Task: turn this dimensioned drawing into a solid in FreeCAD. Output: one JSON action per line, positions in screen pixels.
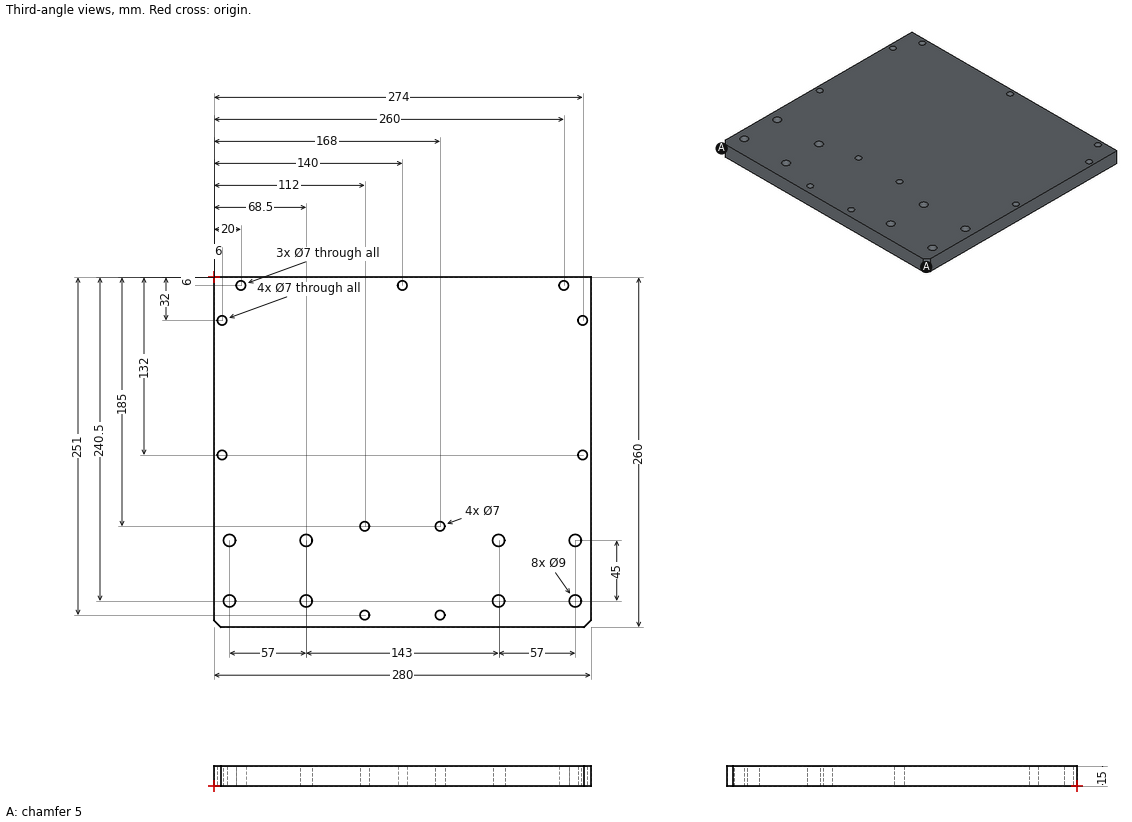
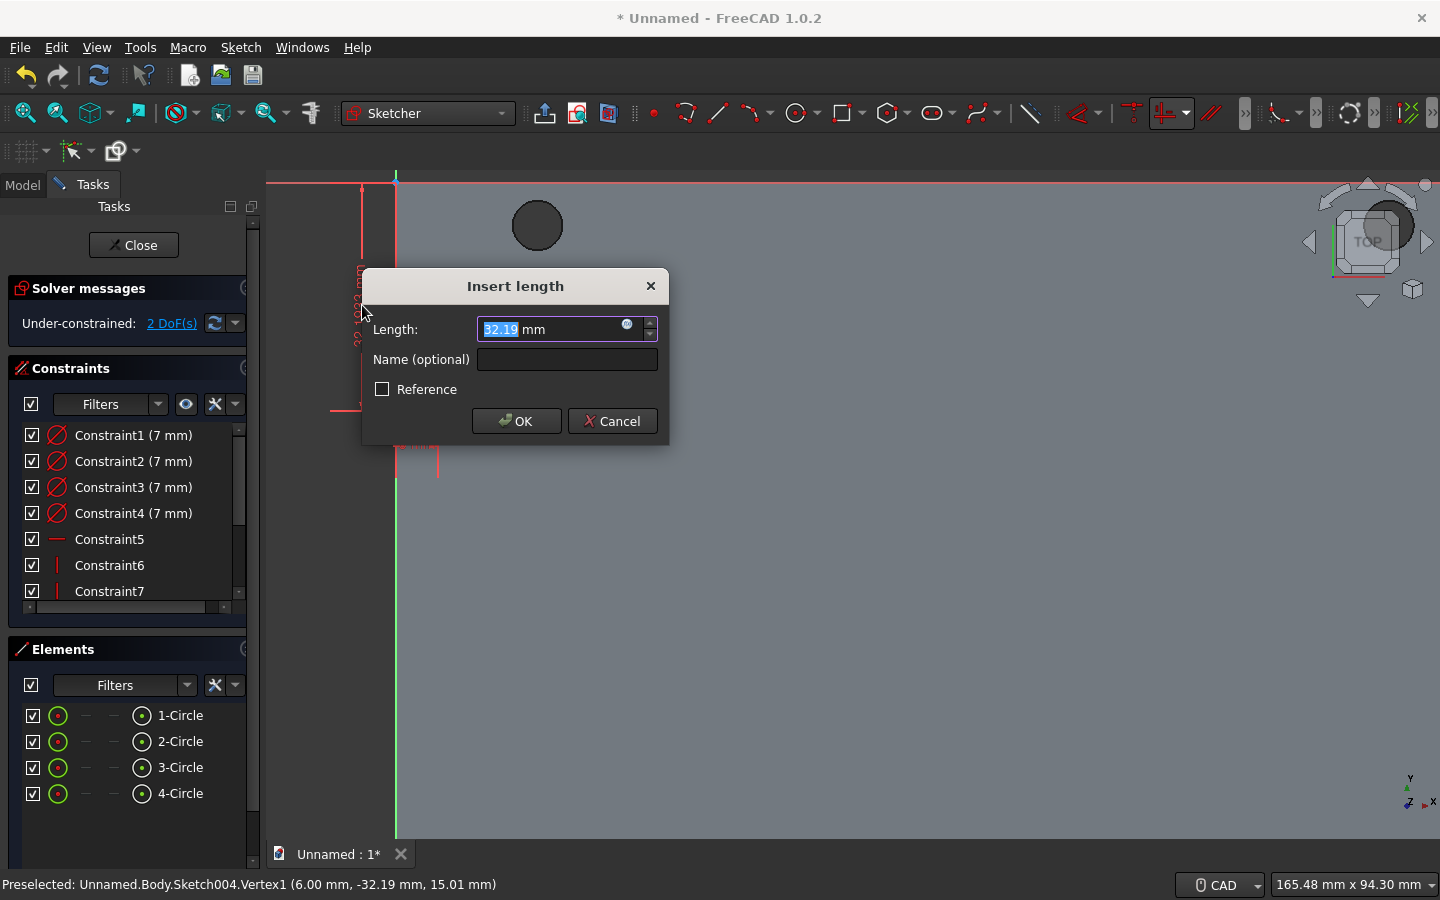
{"action": "type", "text": "32"}
{"action": "key", "text": "Return"}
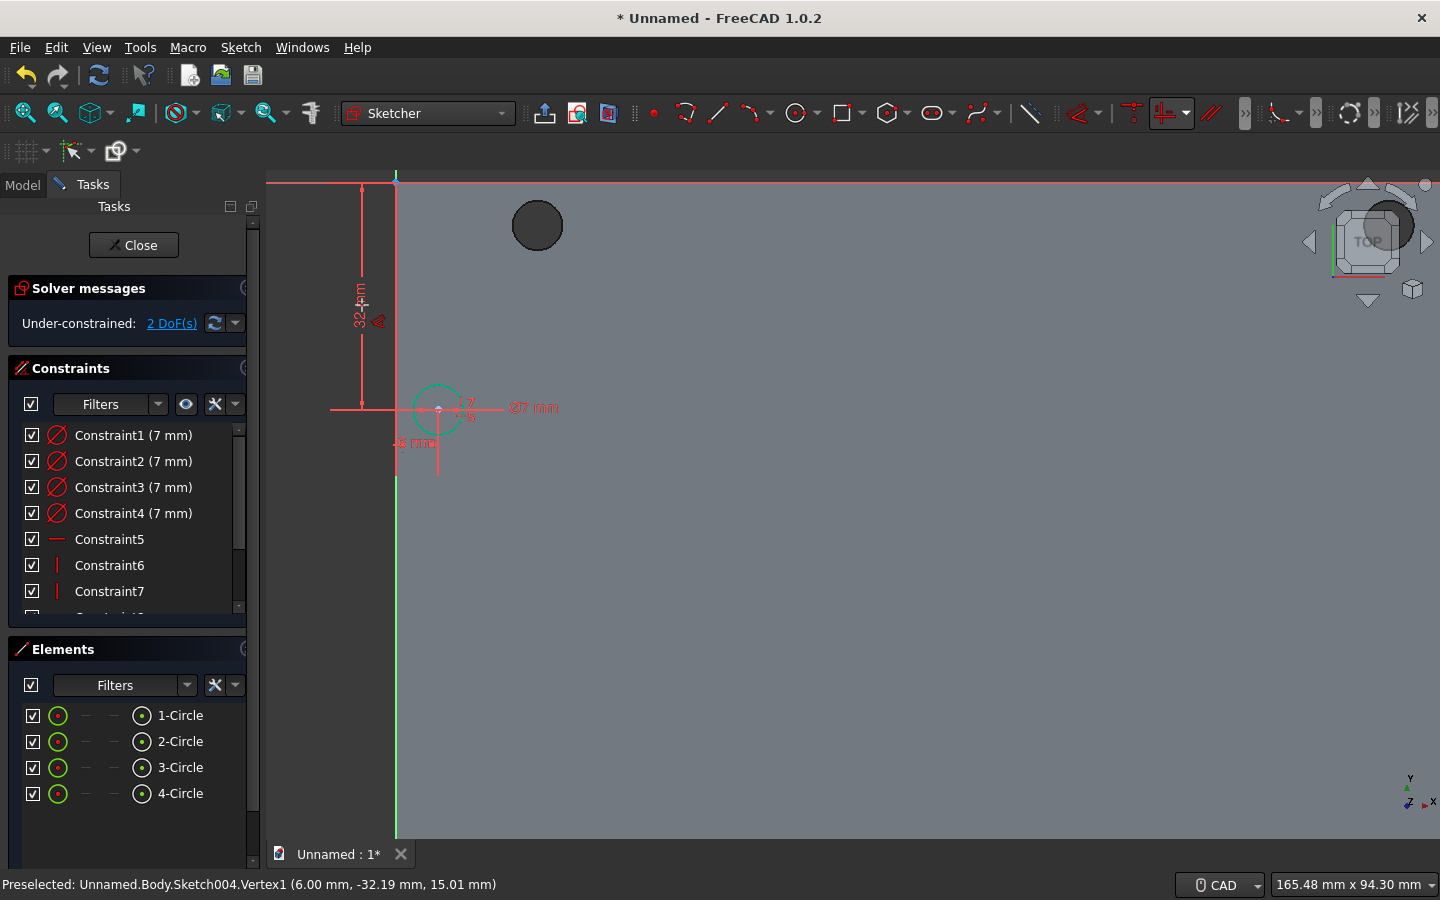
{"action": "scroll", "coordinate": [438, 412], "scroll_direction": "down", "scroll_amount": 5}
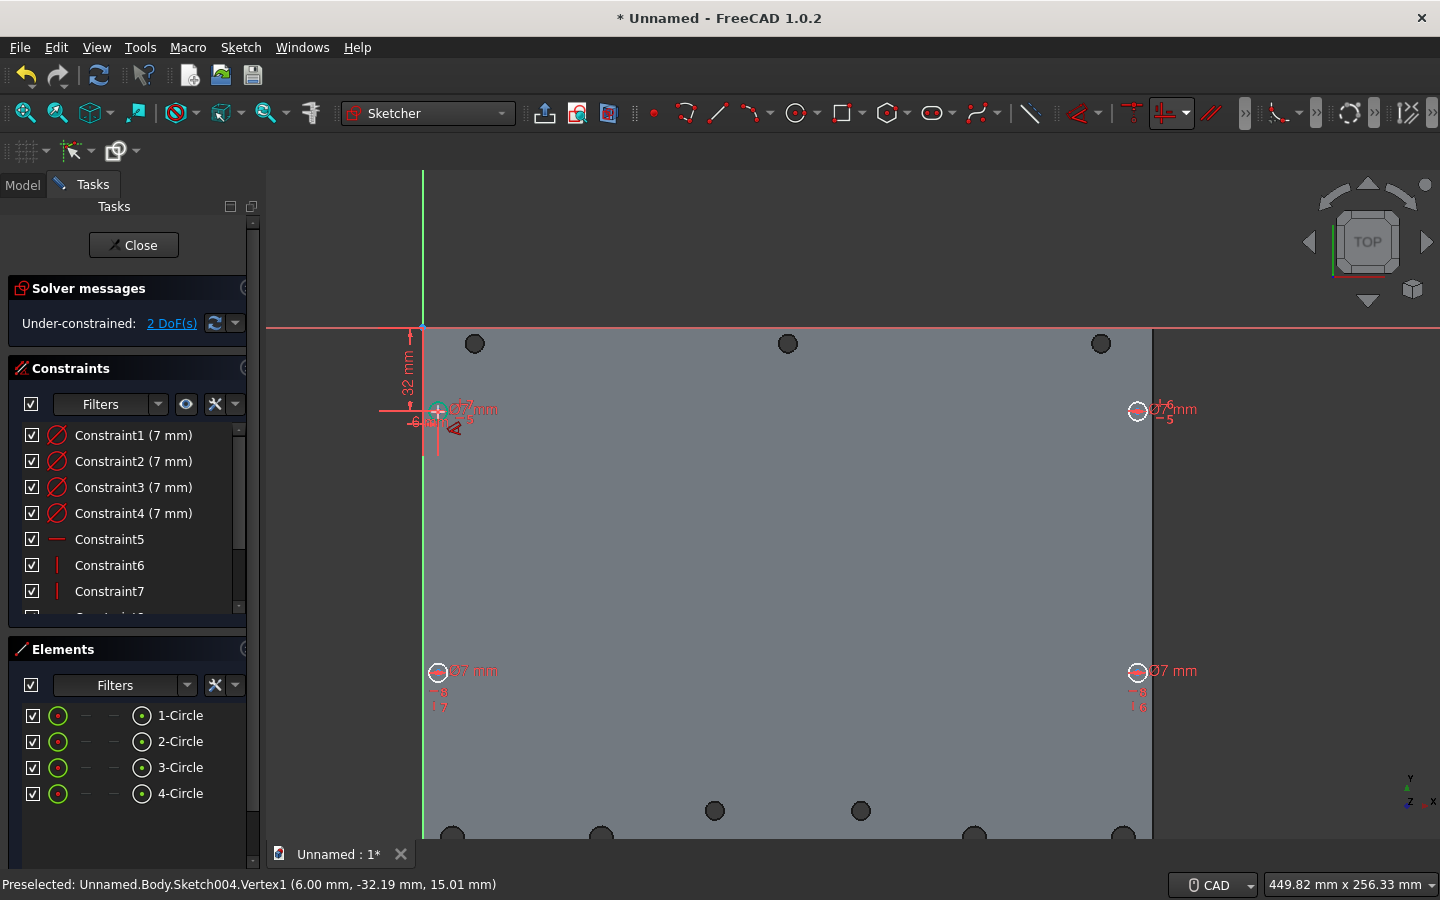
{"action": "left_click", "coordinate": [1138, 411]}
{"action": "left_click", "coordinate": [780, 294]}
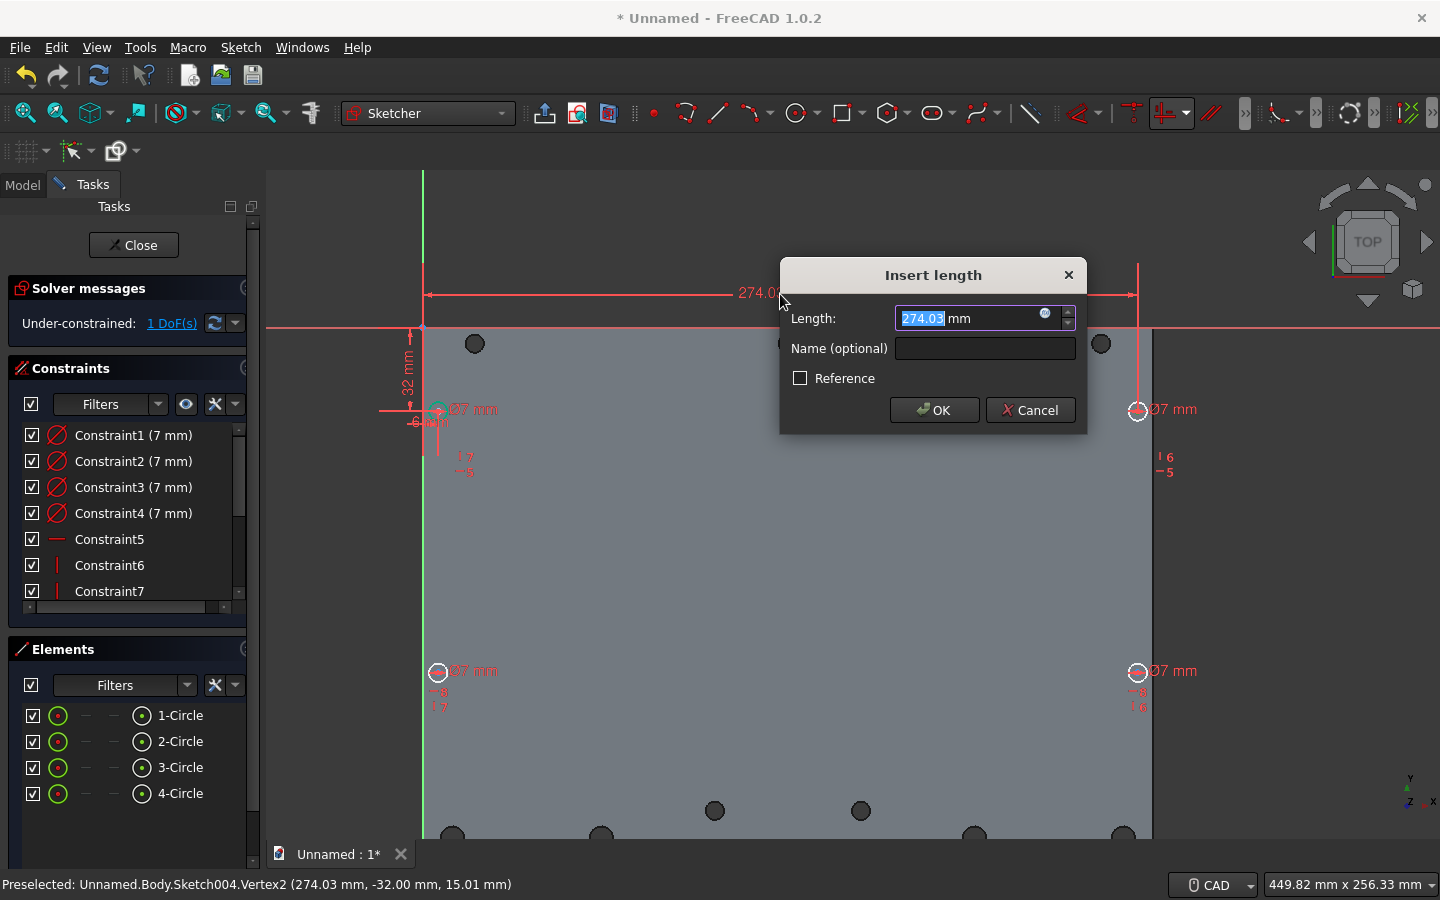
{"action": "type", "text": "274"}
{"action": "key", "text": "Return"}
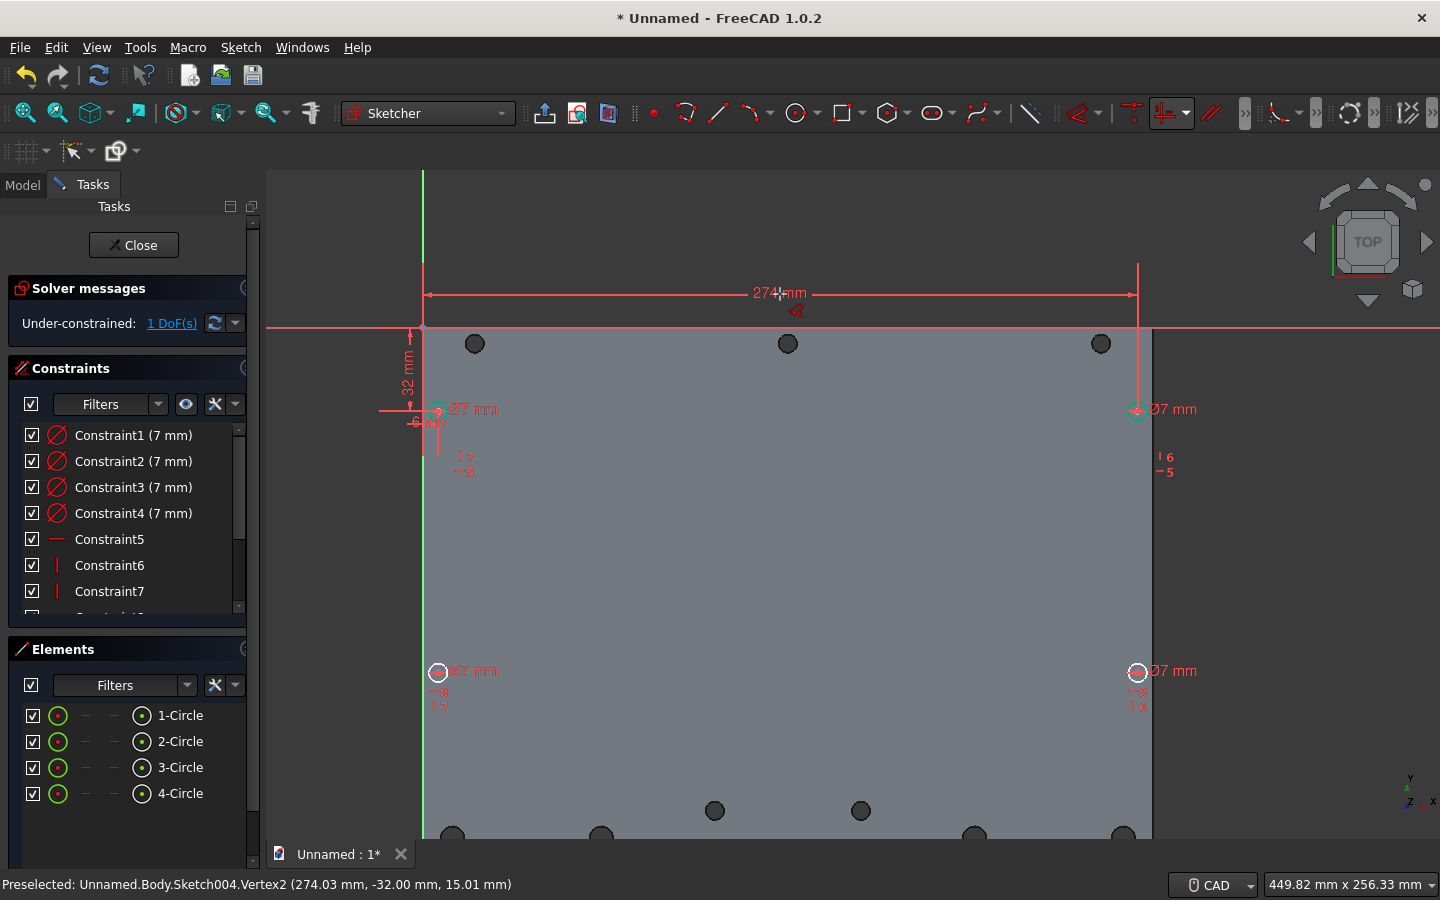
{"action": "left_click", "coordinate": [1138, 673]}
{"action": "left_click", "coordinate": [389, 500]}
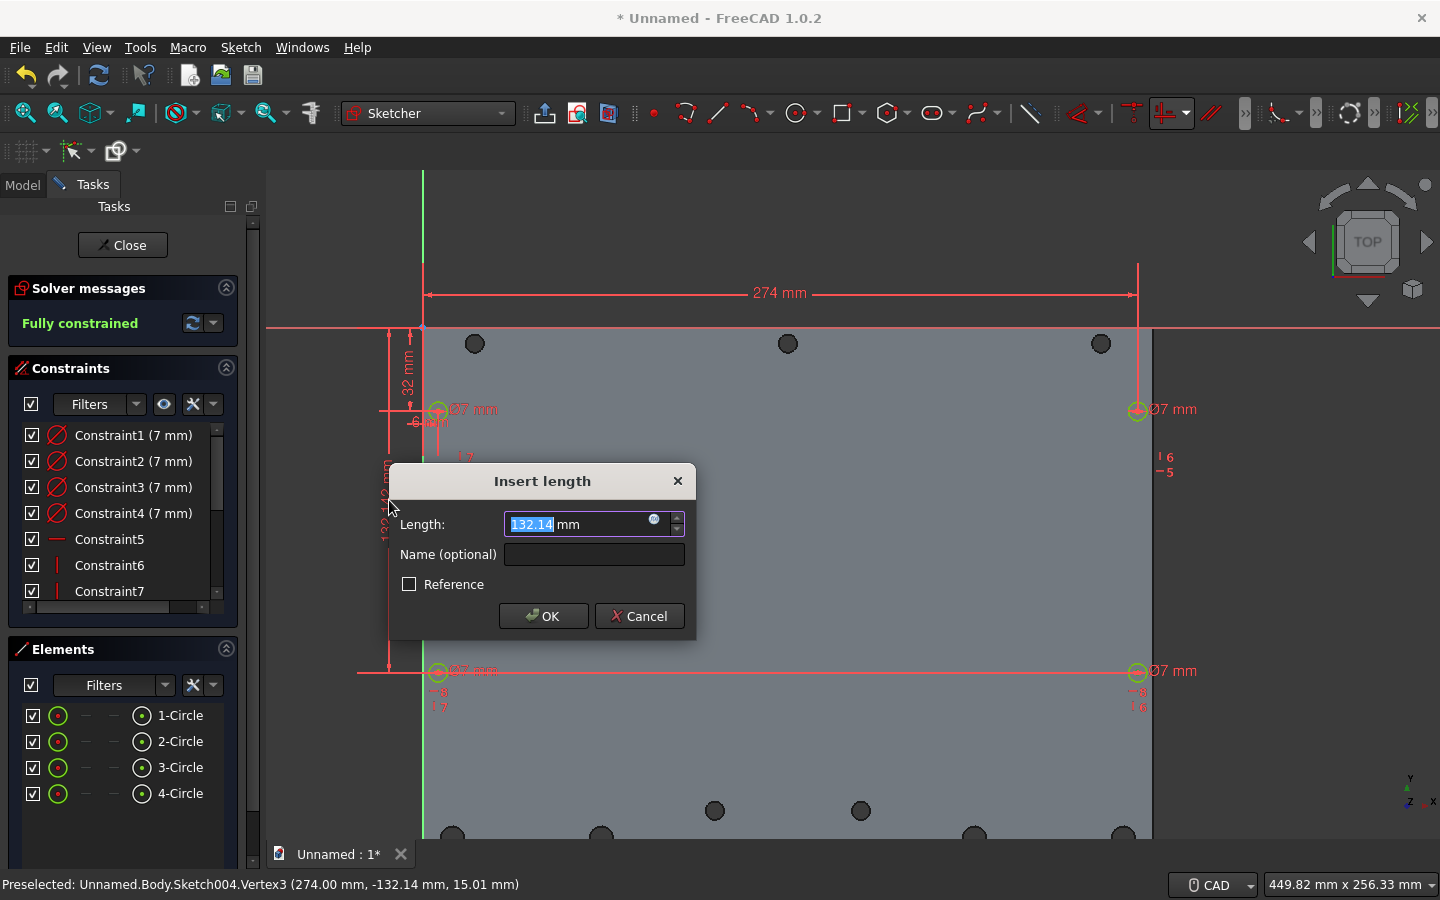
{"action": "type", "text": "132"}
{"action": "key", "text": "Return"}
{"action": "key", "text": "Escape"}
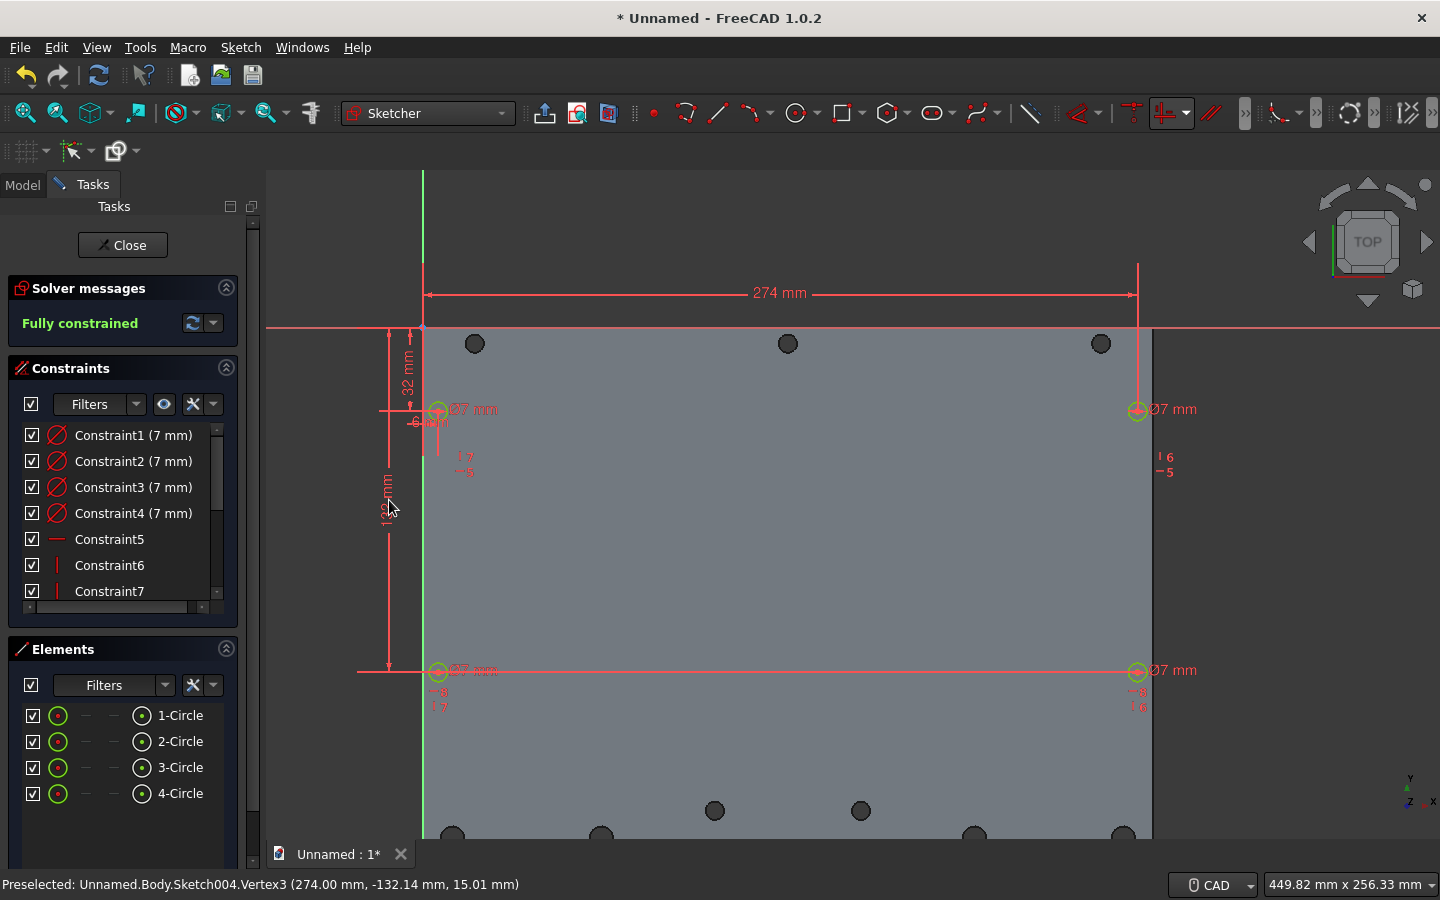
{"action": "left_click", "coordinate": [123, 245]}